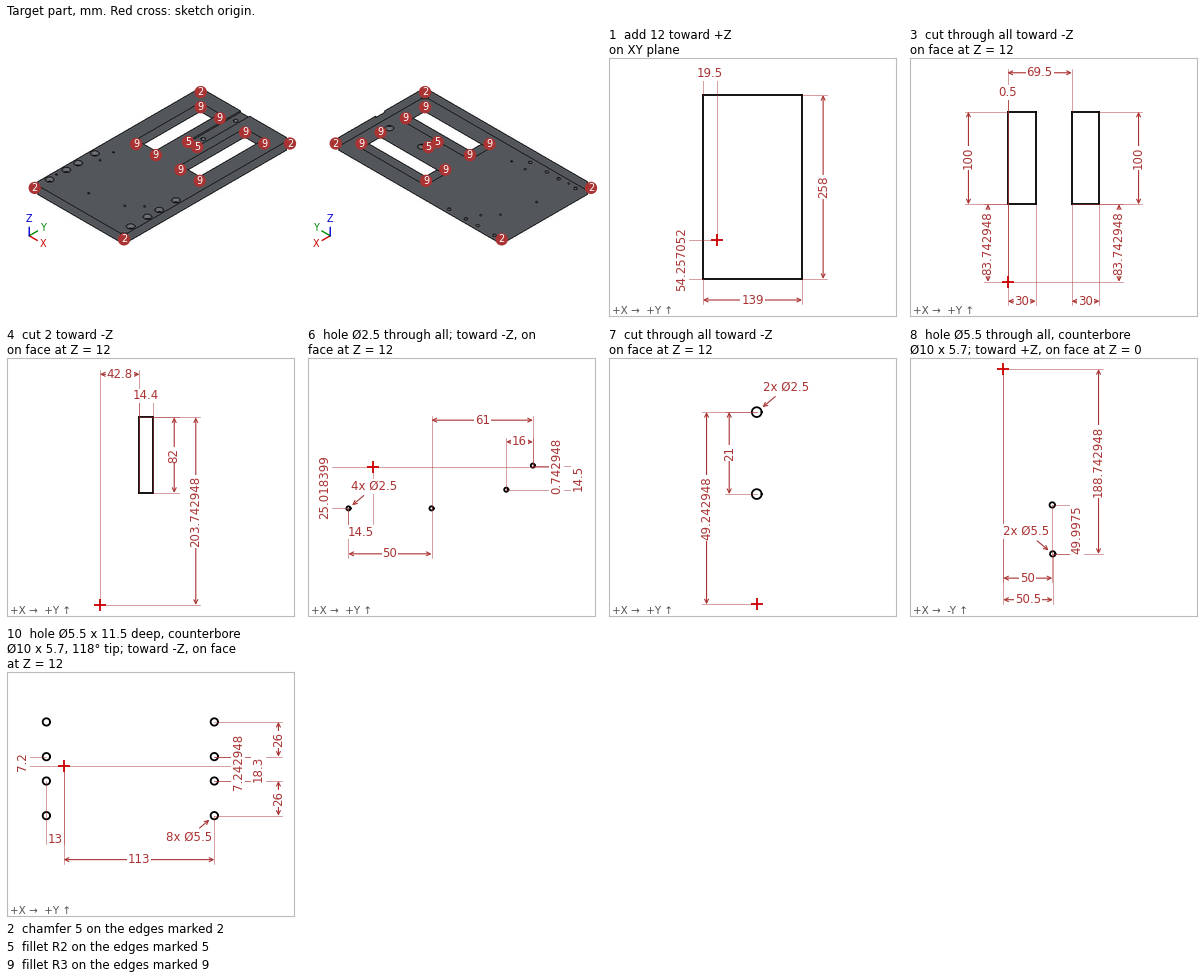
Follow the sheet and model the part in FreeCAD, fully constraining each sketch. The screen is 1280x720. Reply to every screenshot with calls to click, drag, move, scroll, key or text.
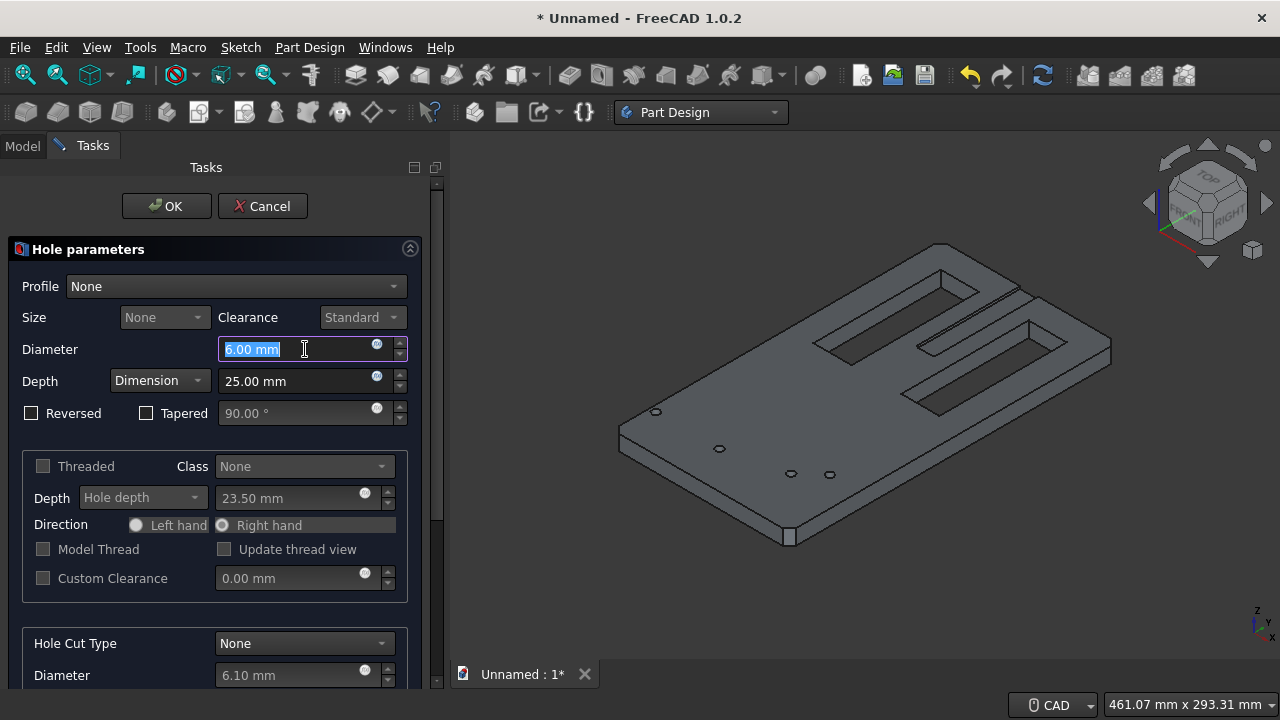
text(2.5)
key(Tab)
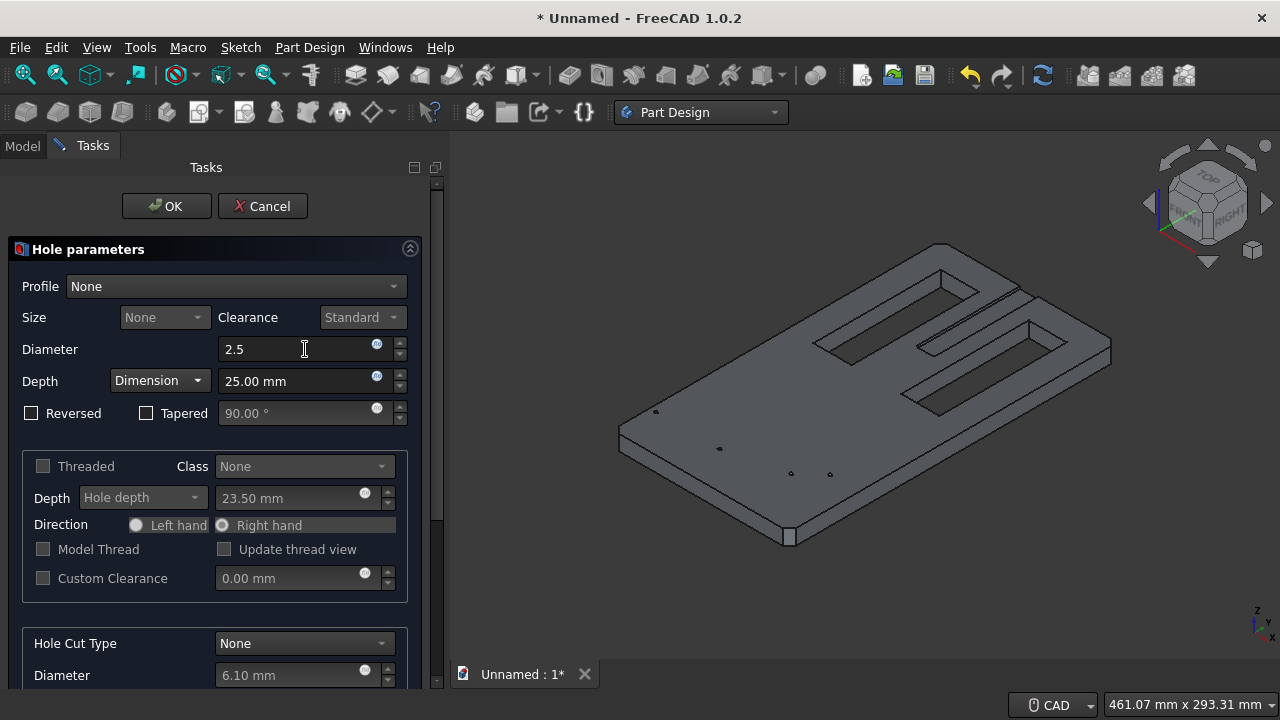
click(161, 380)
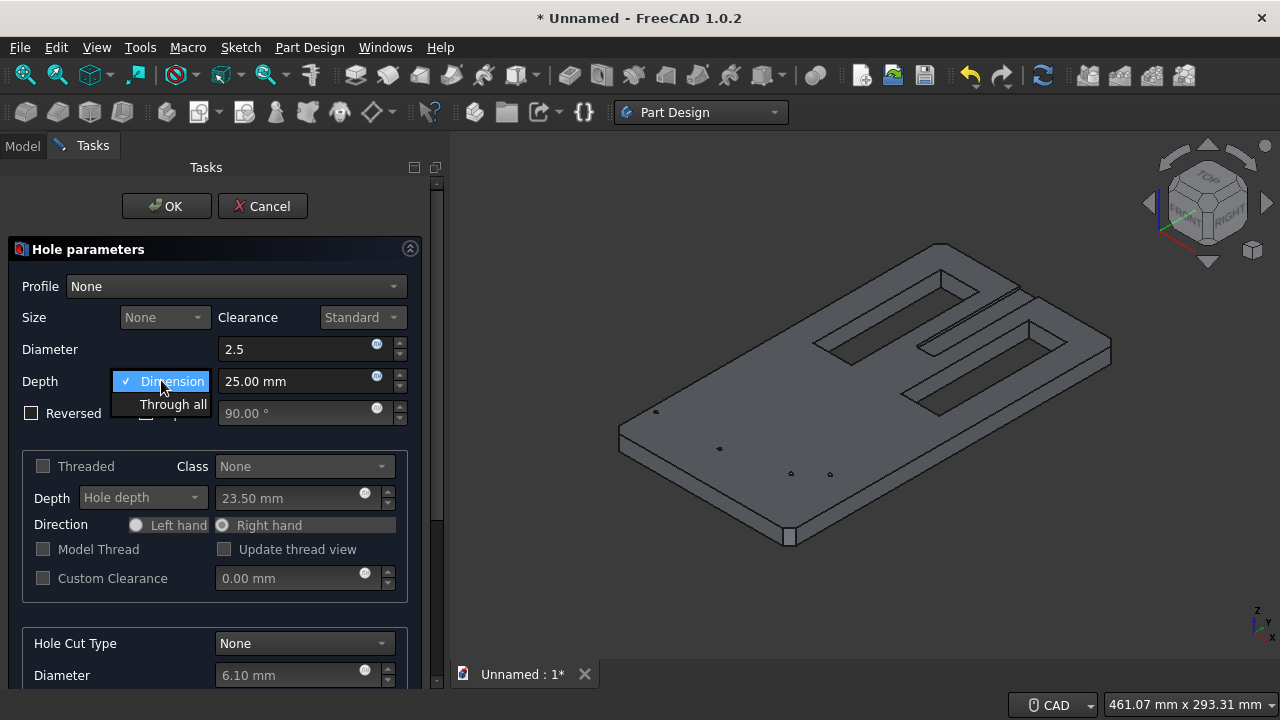
click(160, 404)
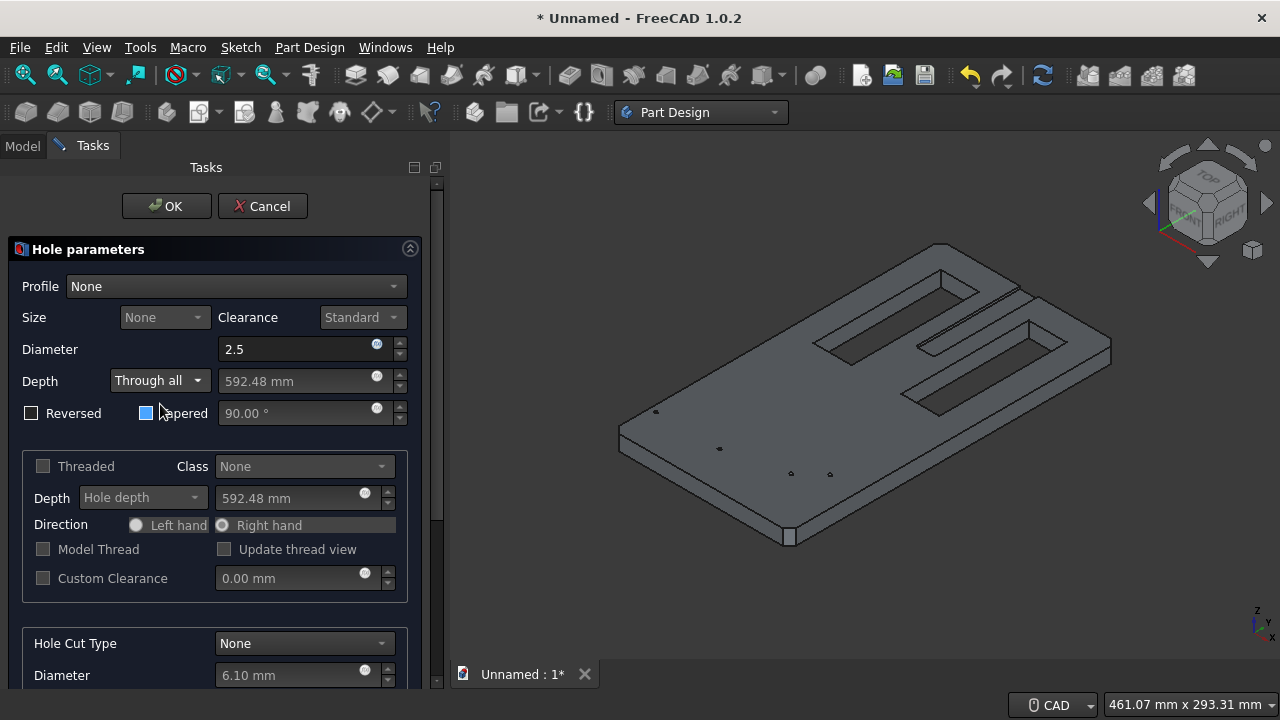
click(167, 206)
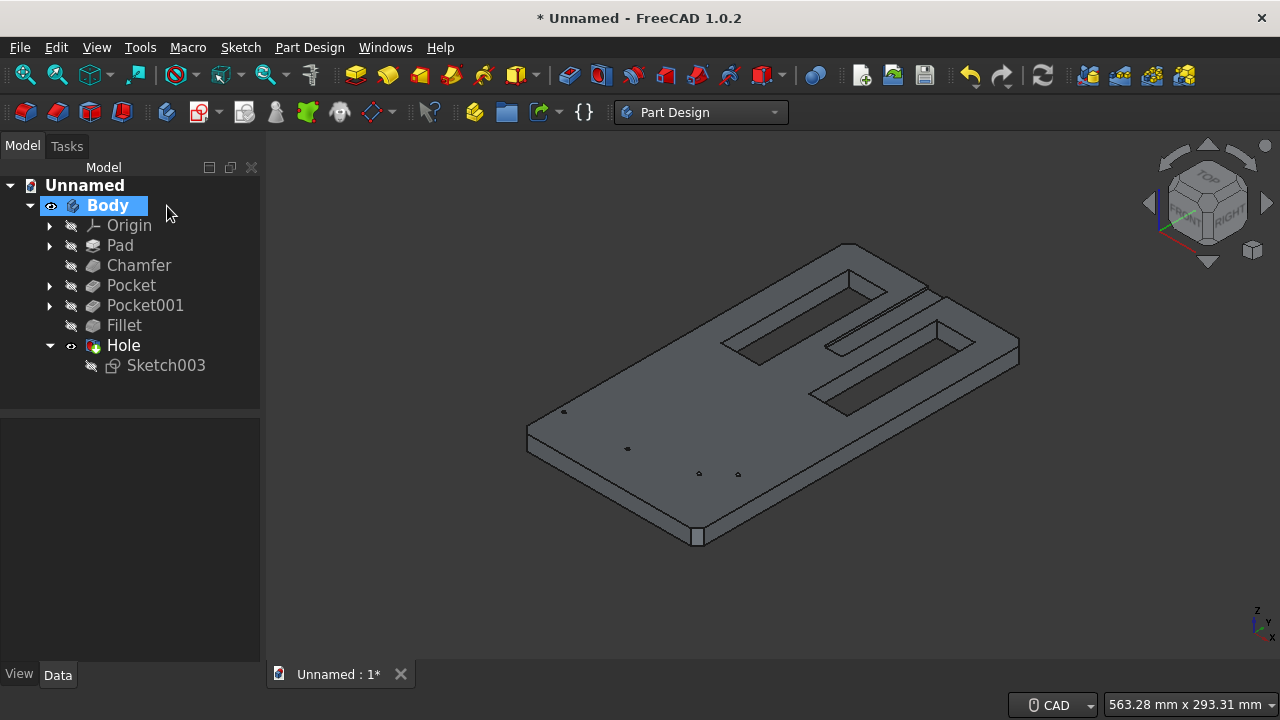
click(726, 412)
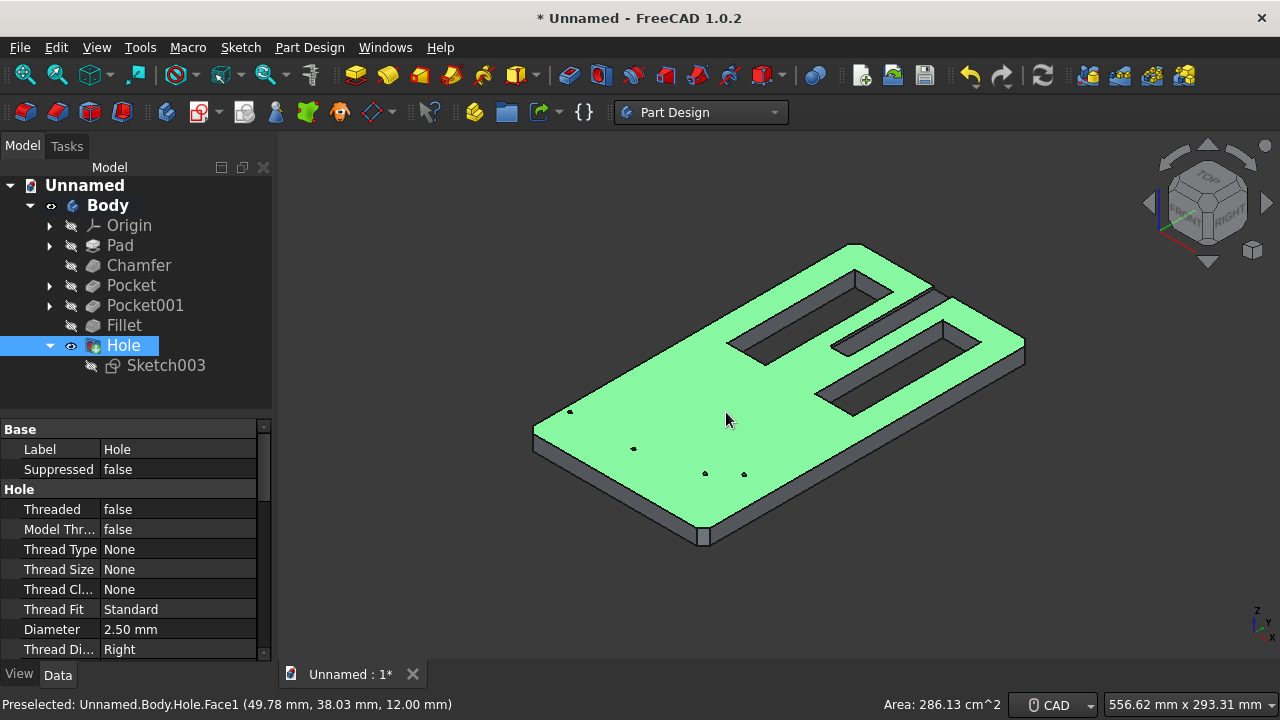
click(200, 112)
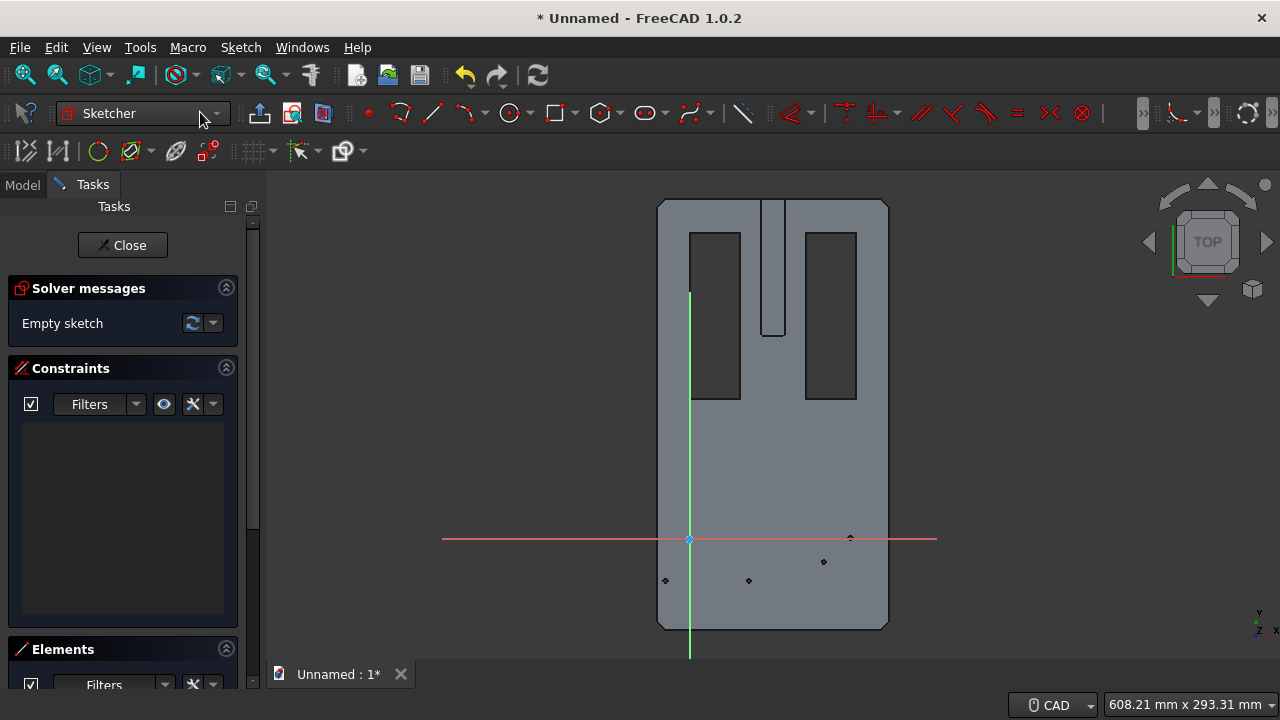
scroll(683, 533, up, 6)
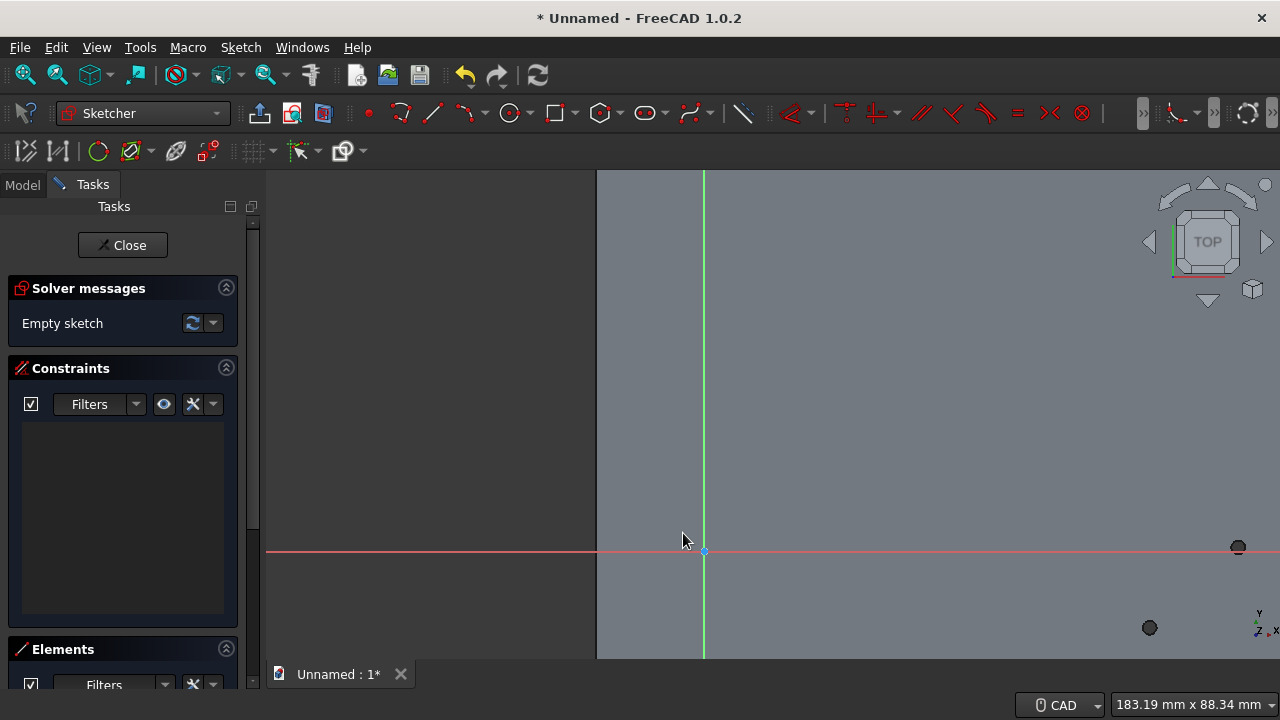
click(510, 114)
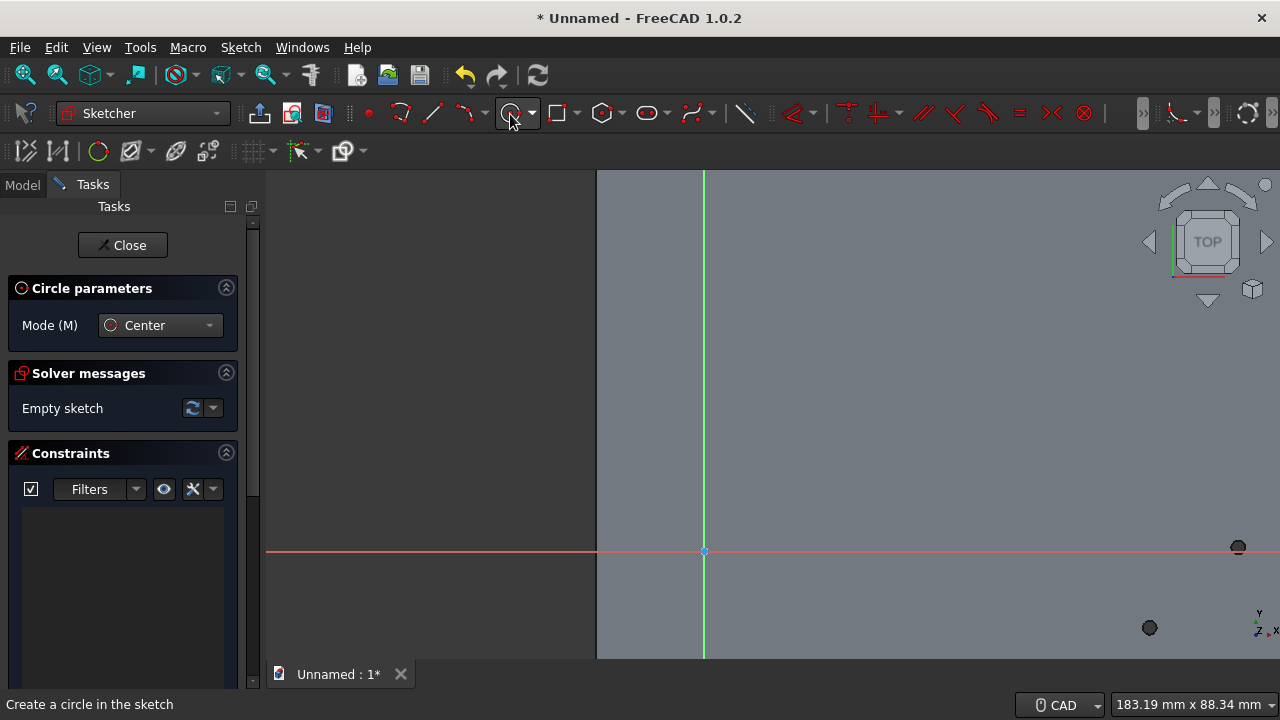
scroll(704, 279, up, 6)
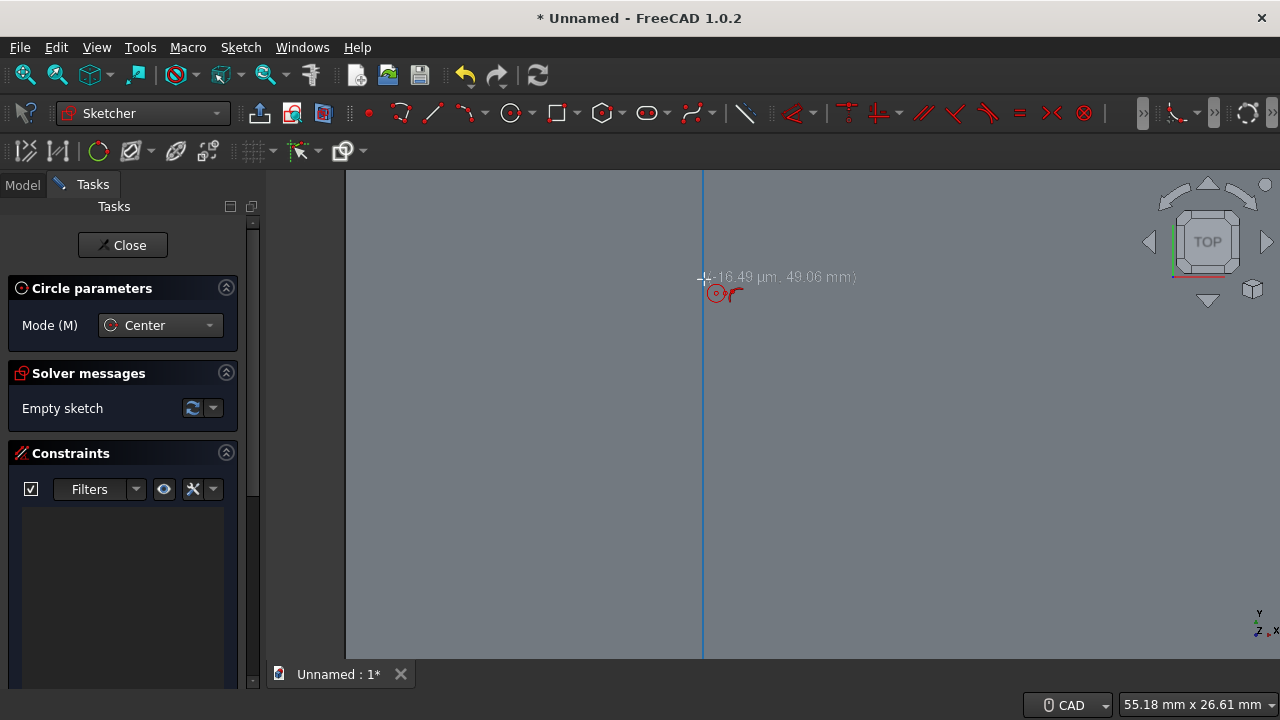
click(703, 278)
move(720, 262)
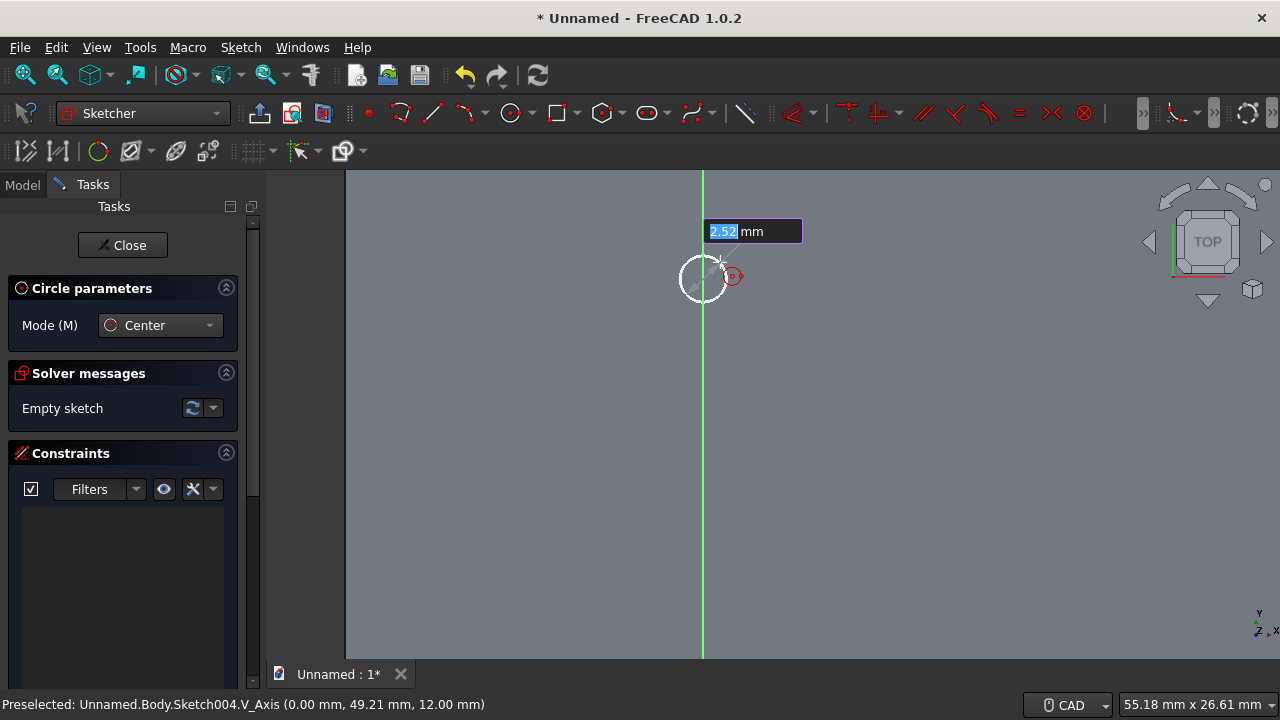
text(2.5)
key(Return)